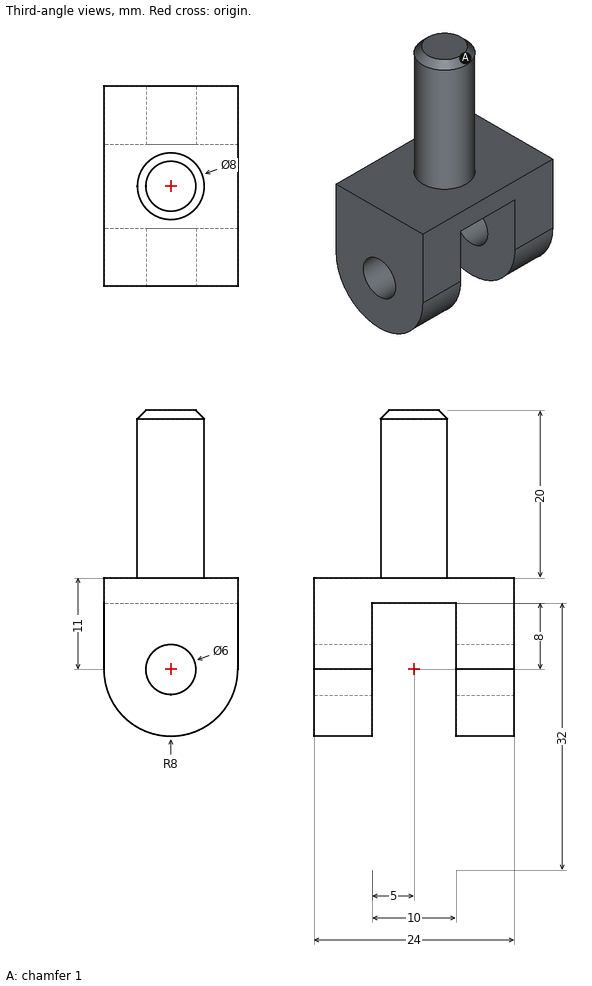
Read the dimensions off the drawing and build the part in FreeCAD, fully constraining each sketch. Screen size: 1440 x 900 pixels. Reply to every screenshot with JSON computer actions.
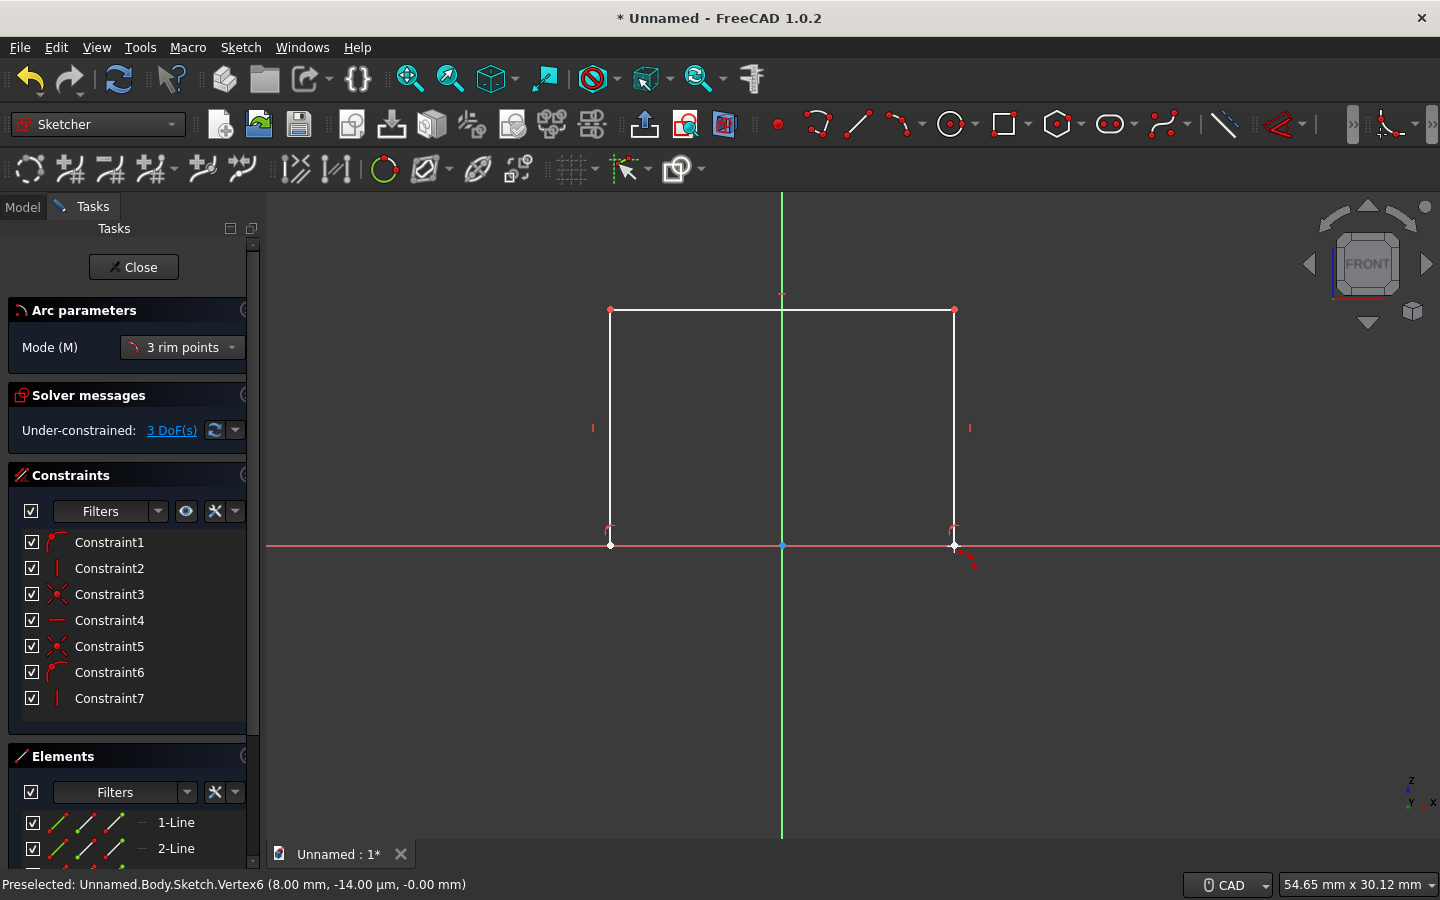
{"action": "left_click", "coordinate": [954, 546]}
{"action": "left_click", "coordinate": [610, 546]}
{"action": "left_click", "coordinate": [729, 709]}
{"action": "key", "text": "Escape"}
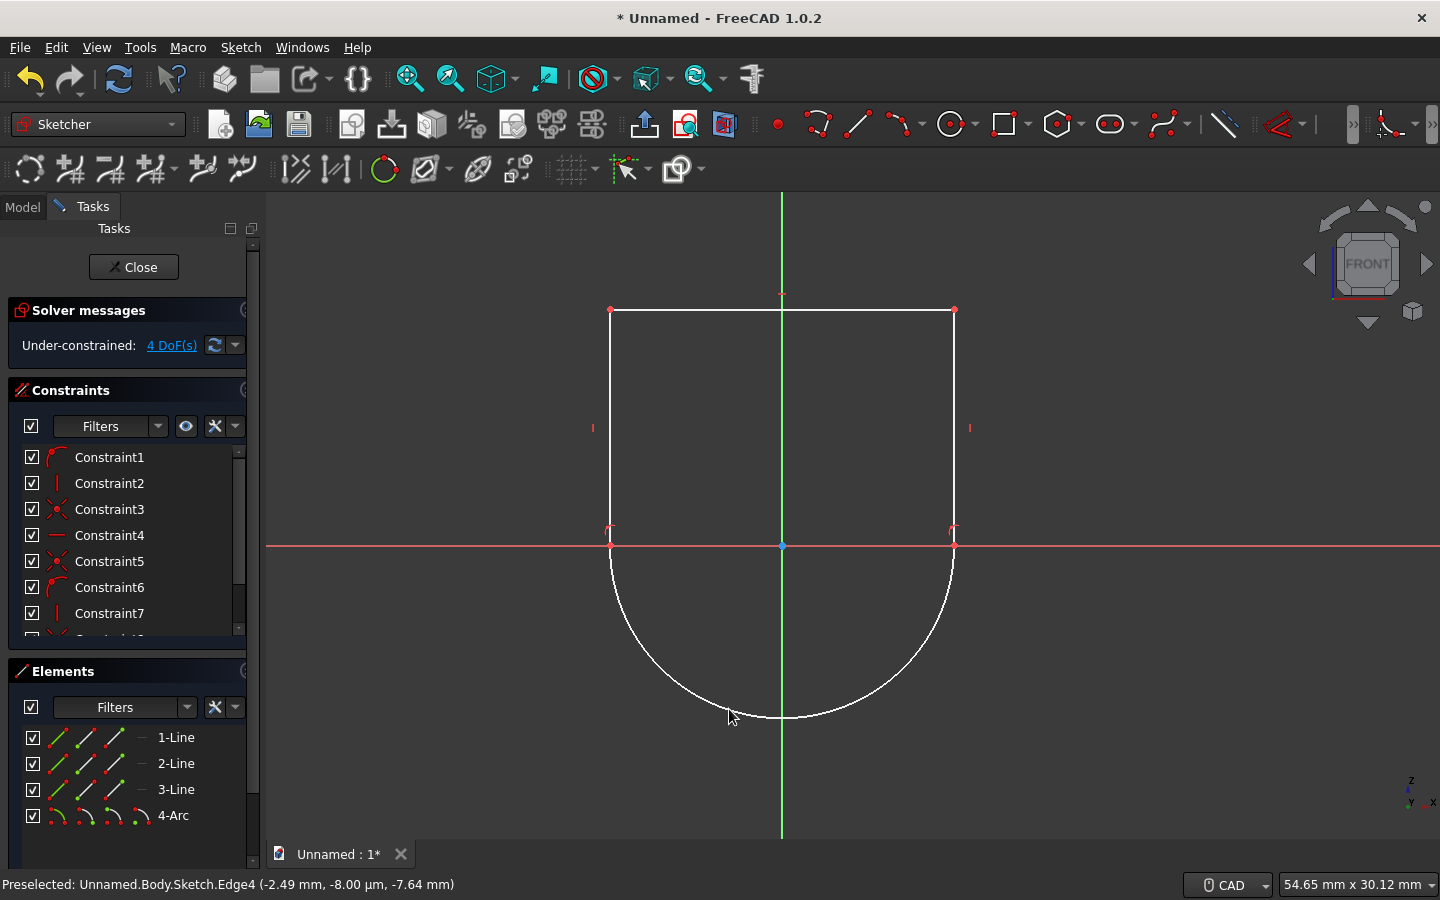
{"action": "left_click", "coordinate": [610, 475]}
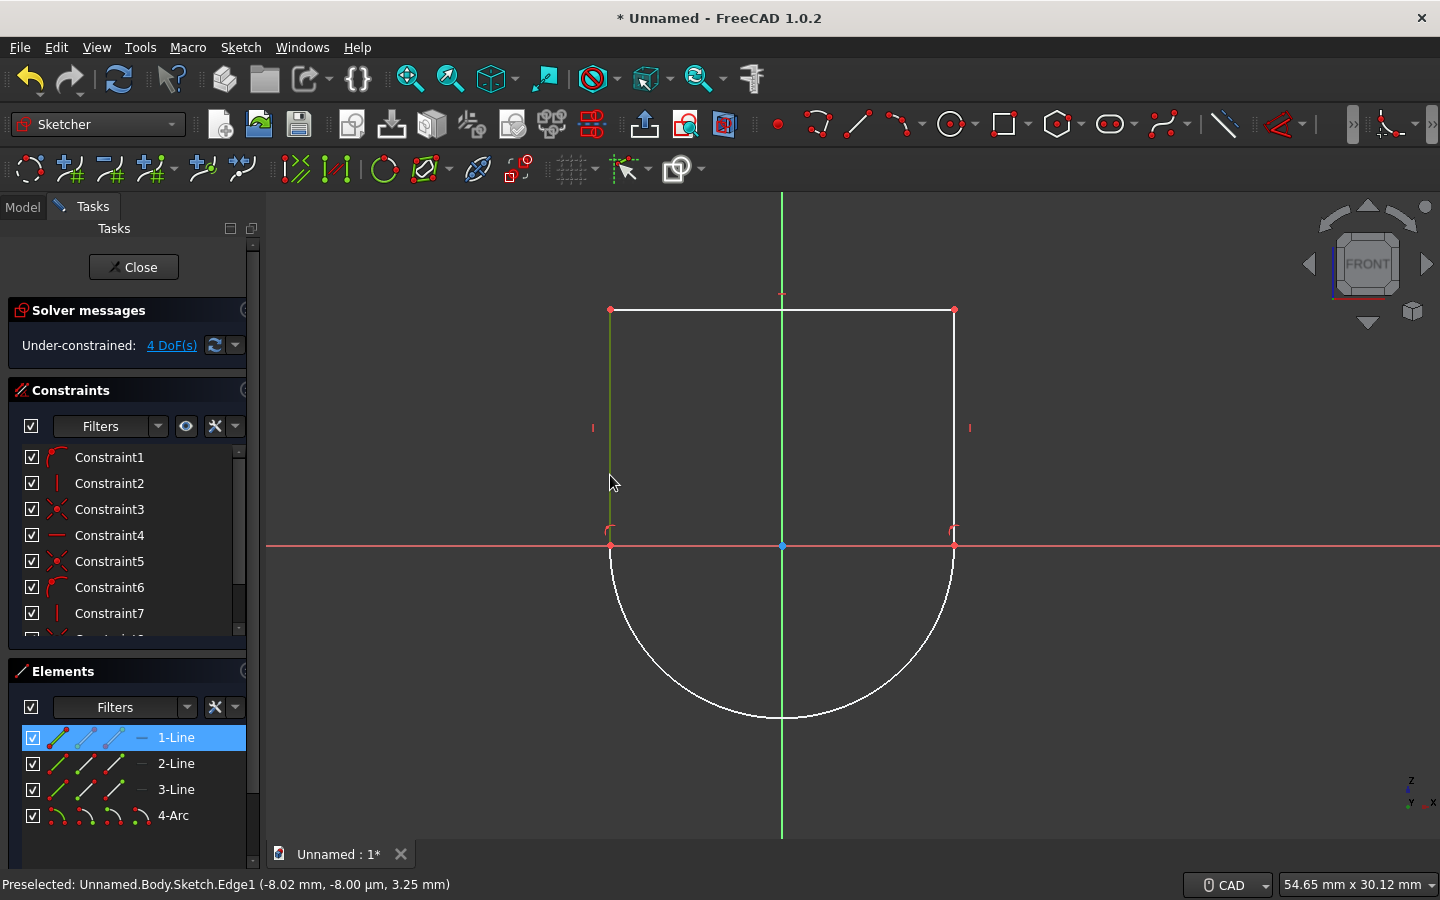
{"action": "left_click", "coordinate": [681, 685]}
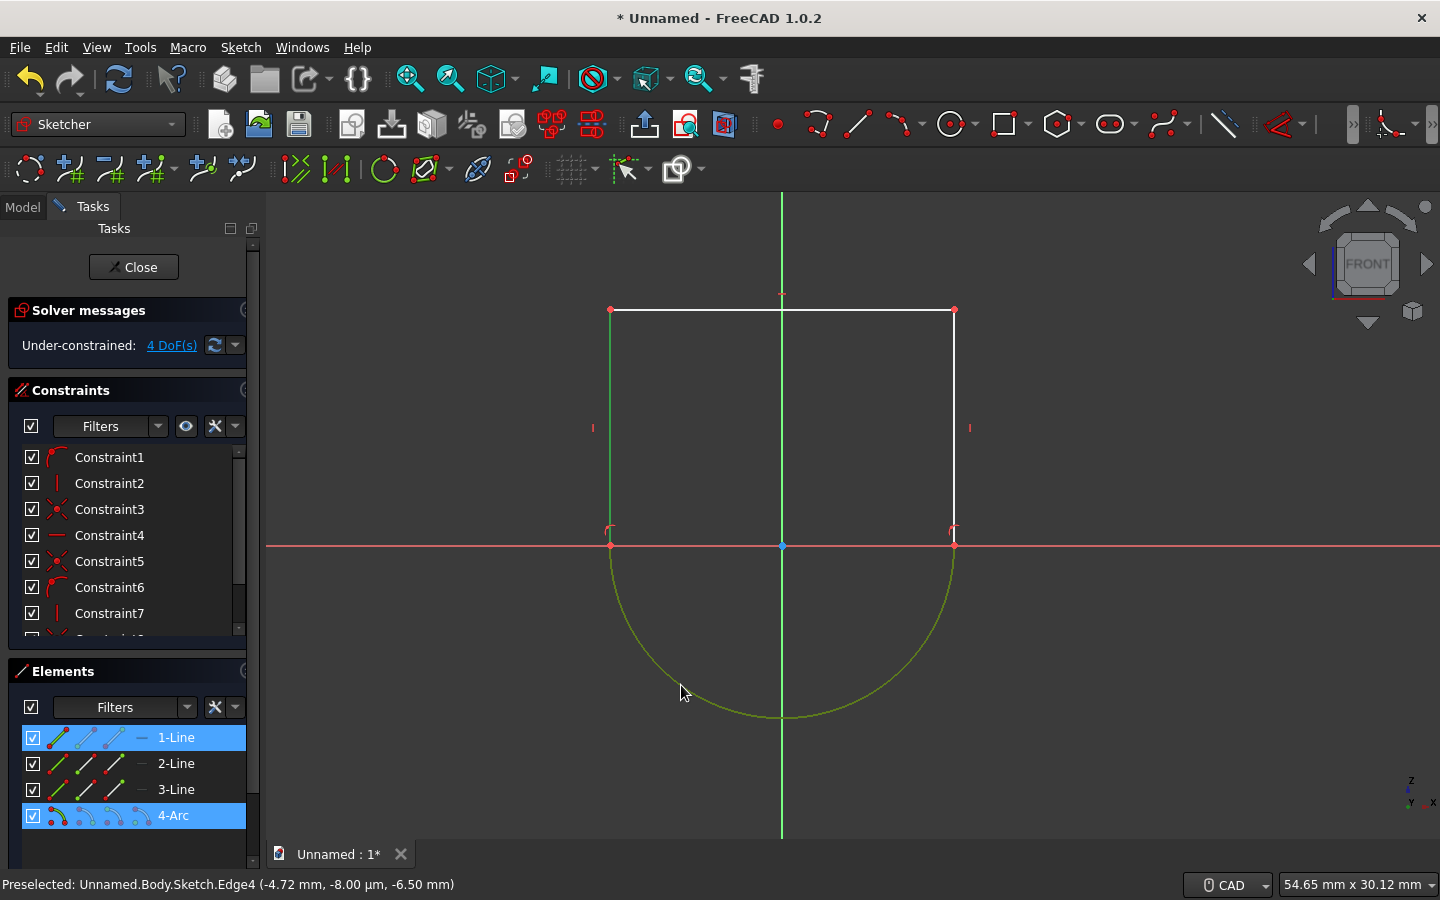
{"action": "key", "text": "t"}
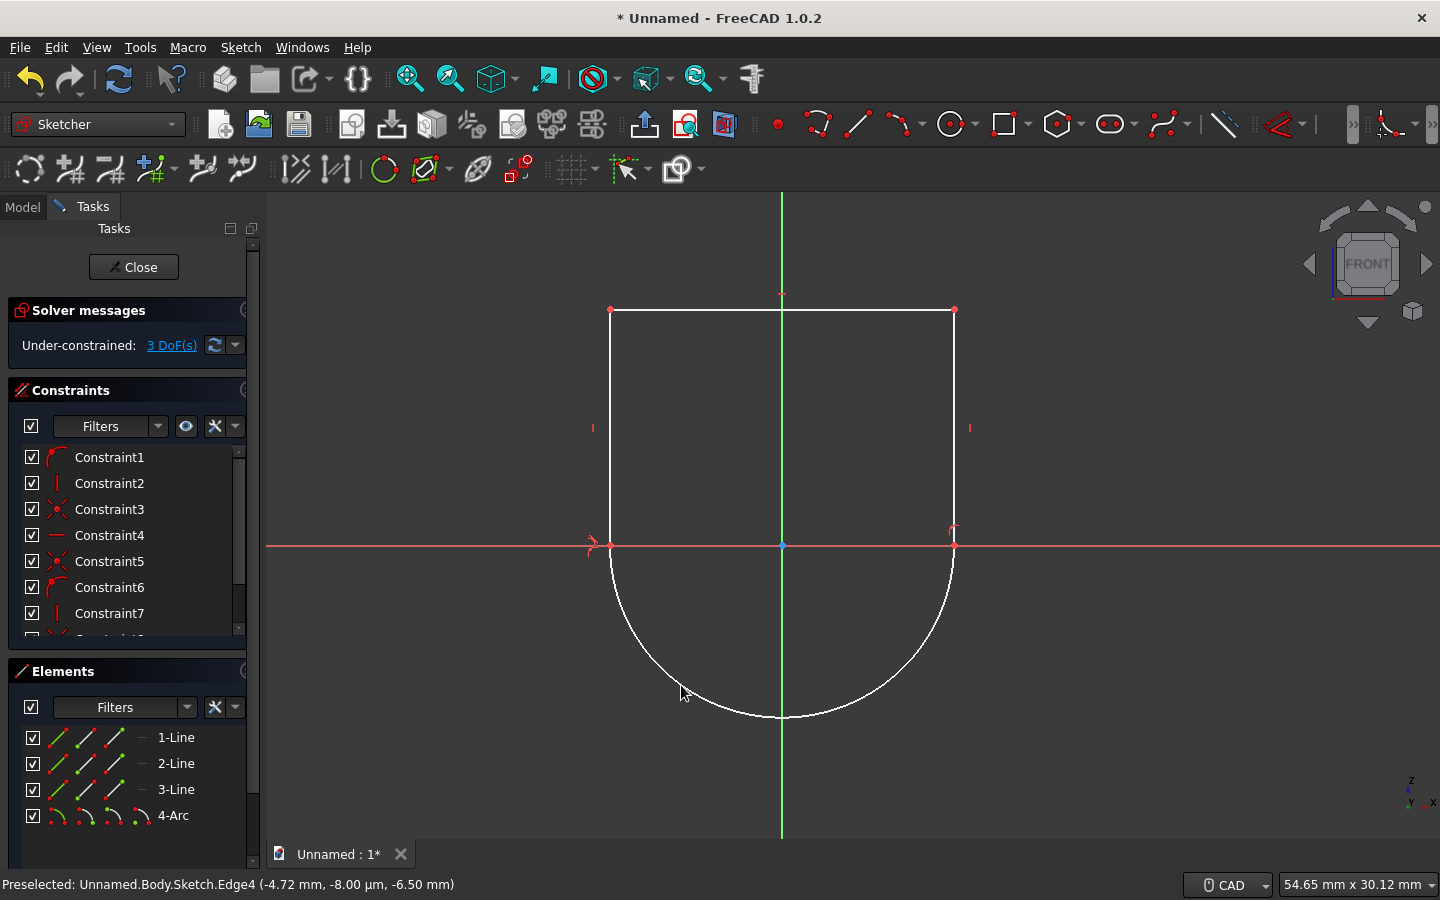
{"action": "left_click", "coordinate": [782, 546]}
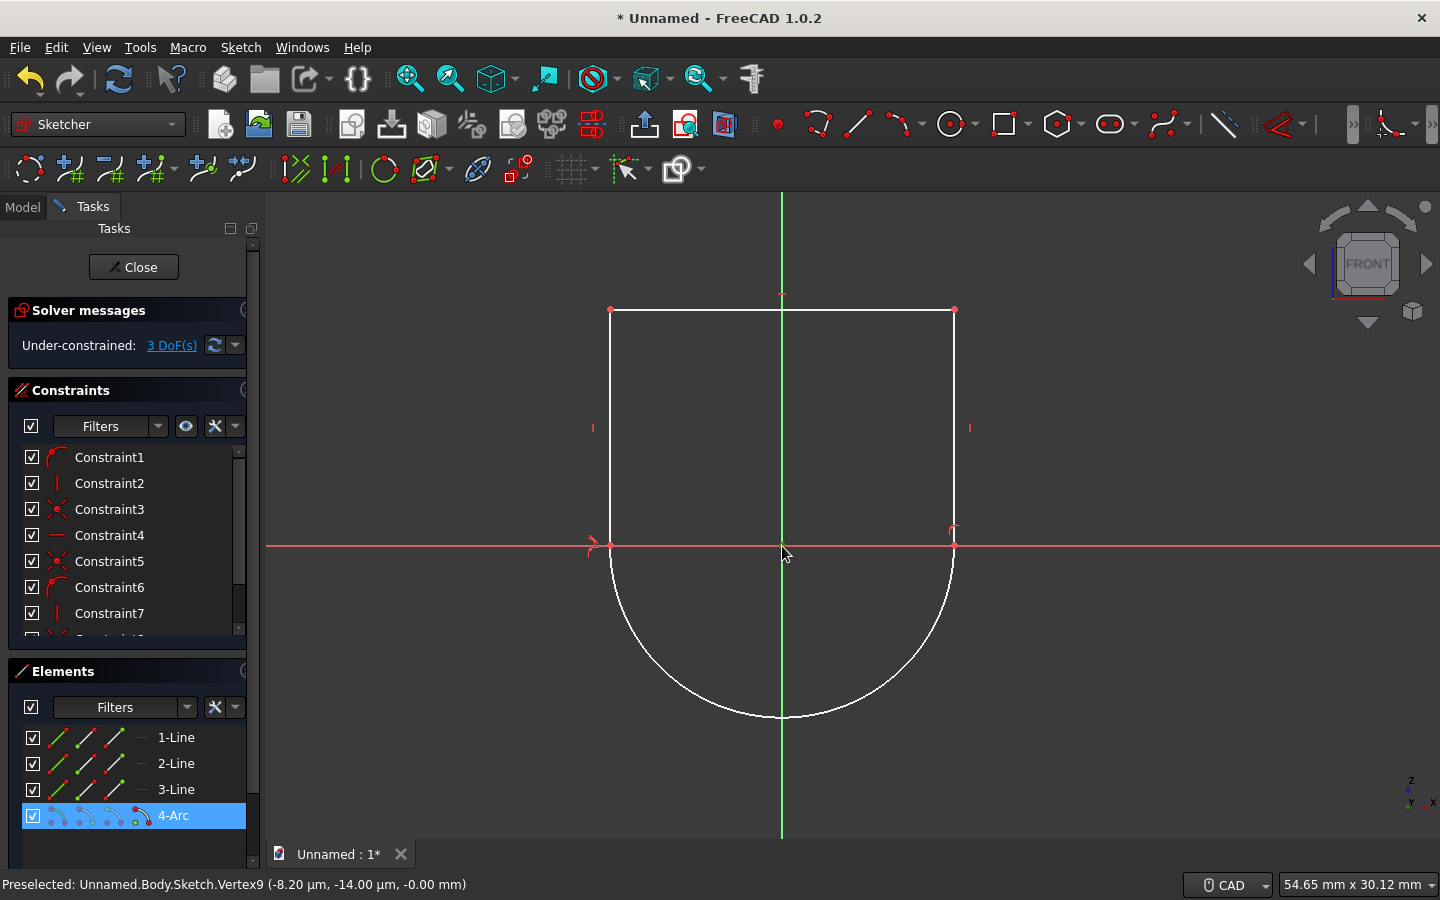
{"action": "left_click", "coordinate": [782, 769]}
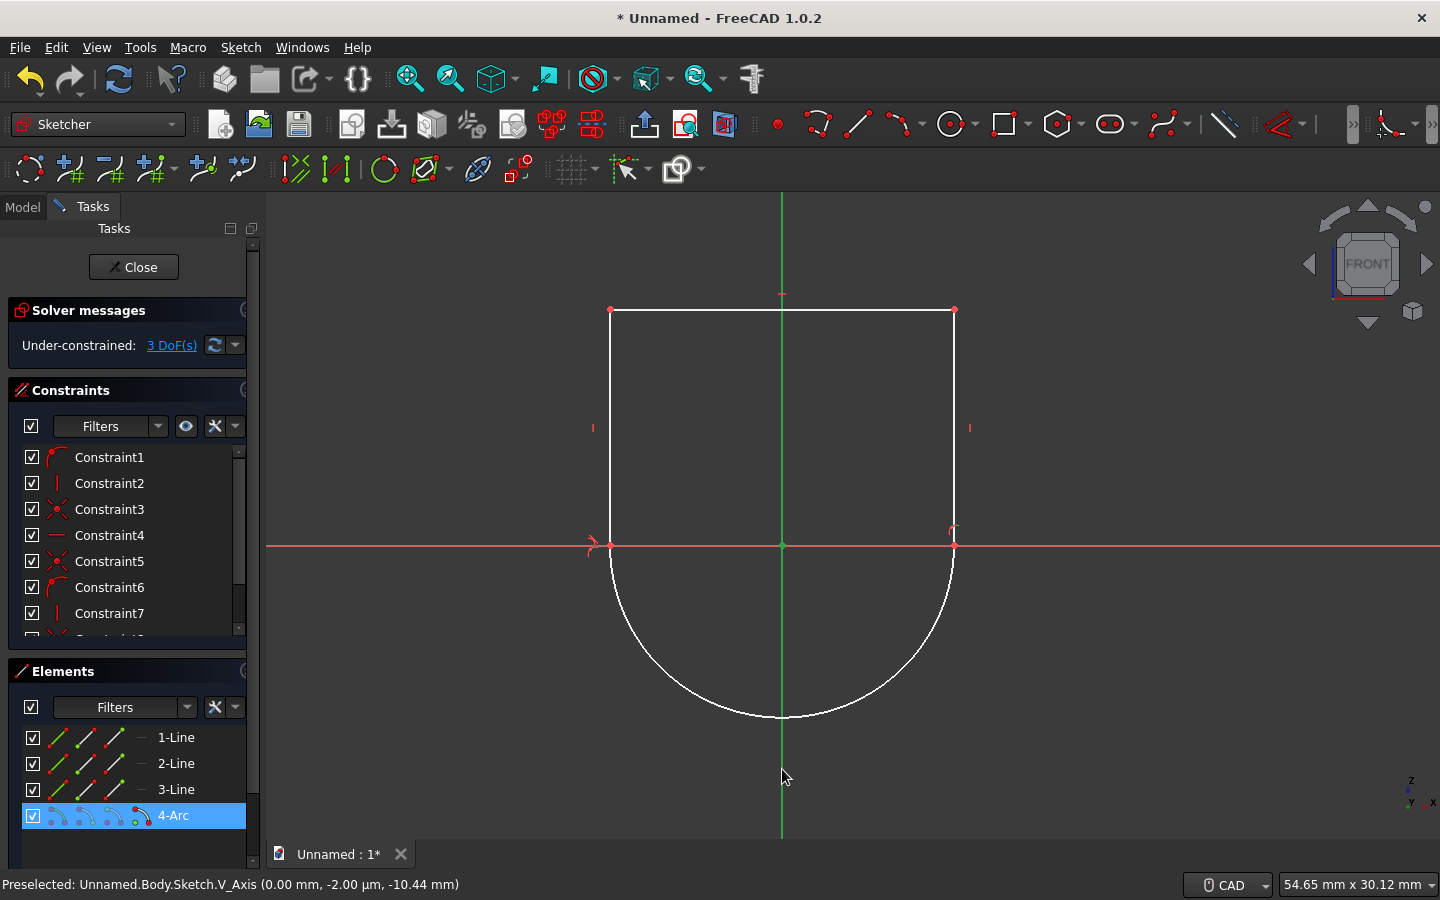
{"action": "key", "text": "c"}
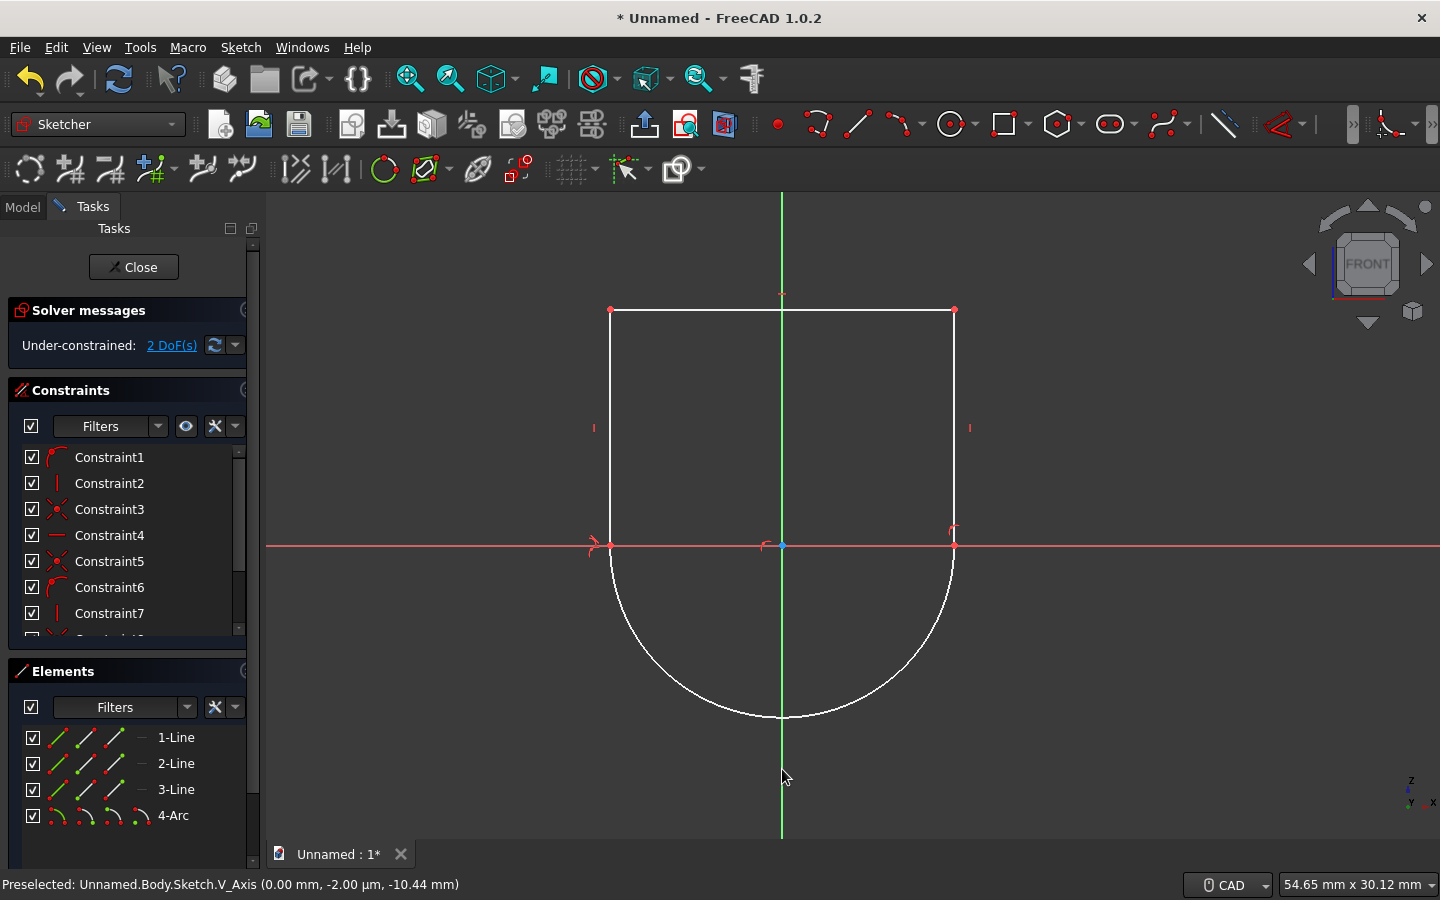
{"action": "left_click", "coordinate": [681, 685]}